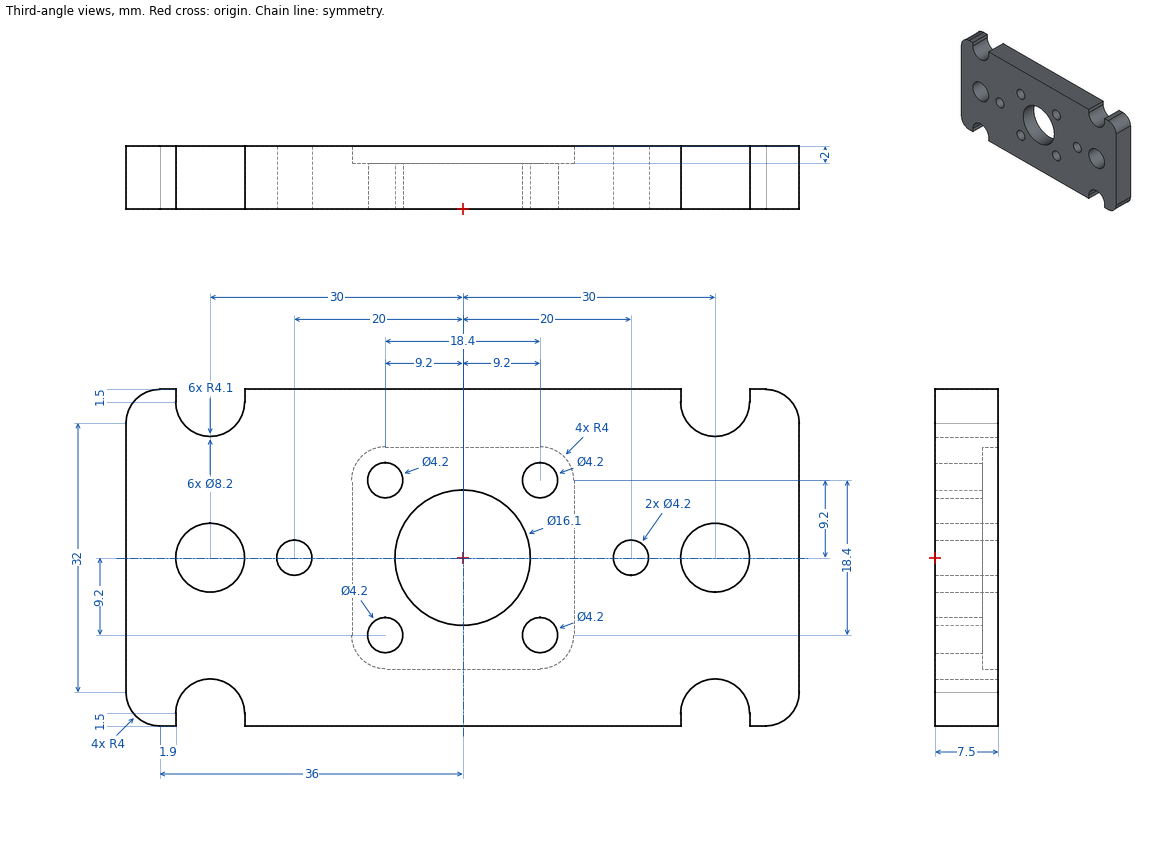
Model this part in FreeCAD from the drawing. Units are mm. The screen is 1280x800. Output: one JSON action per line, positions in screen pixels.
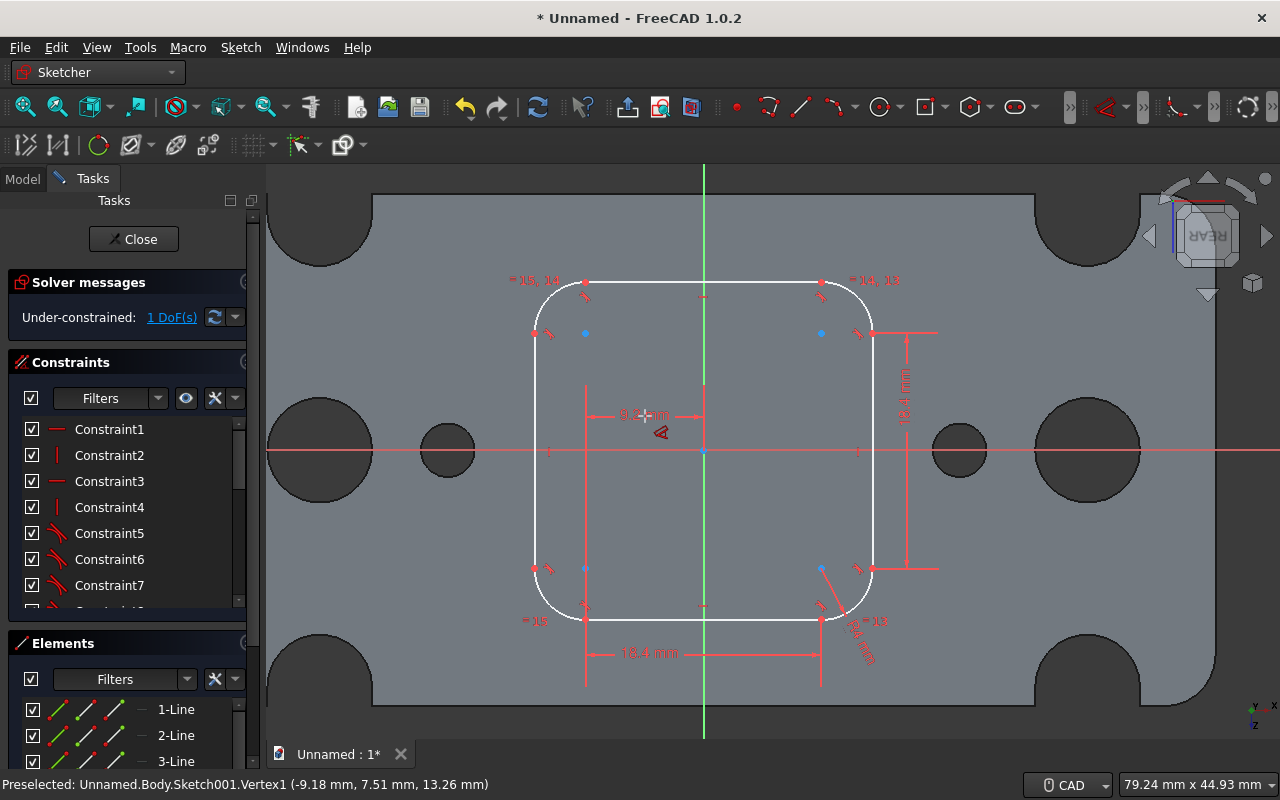
{"action": "left_click", "coordinate": [873, 569]}
{"action": "left_click", "coordinate": [907, 510]}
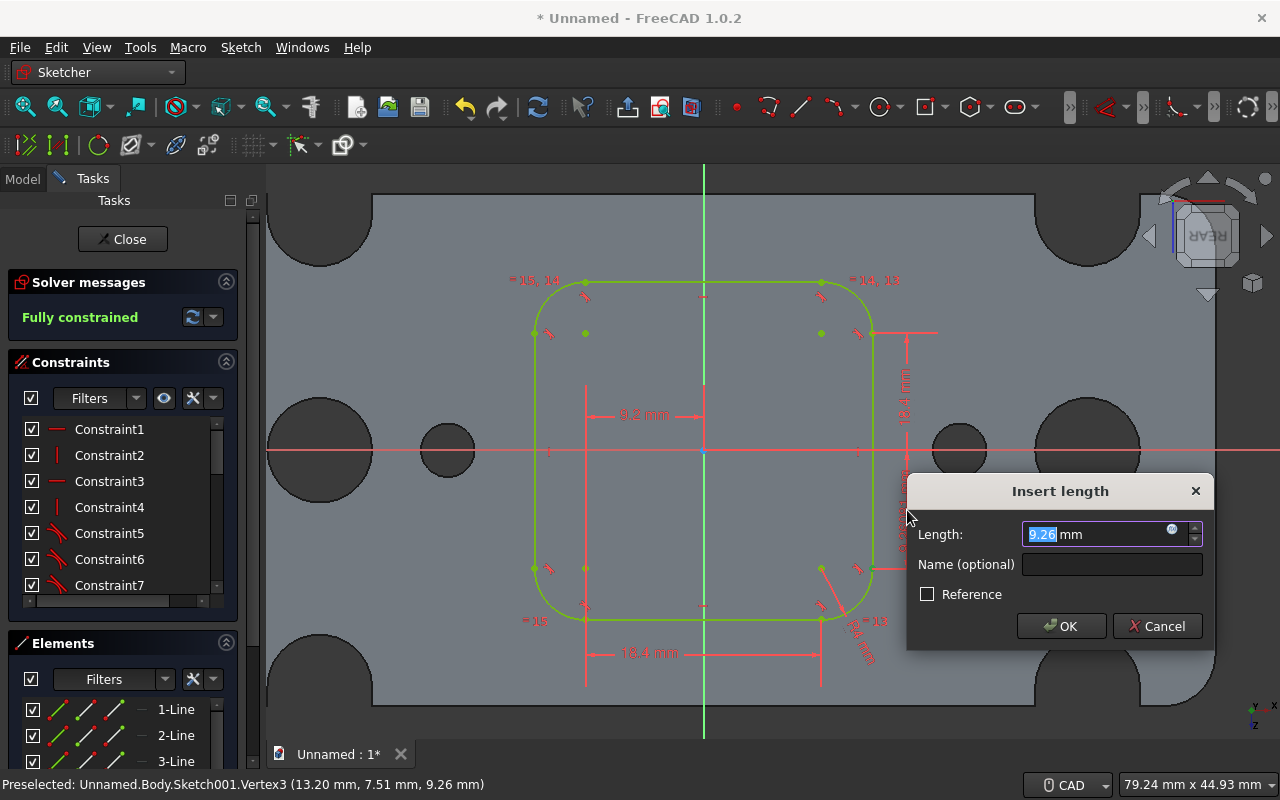
{"action": "type", "text": "9.2"}
{"action": "key", "text": "Return"}
{"action": "key", "text": "Escape"}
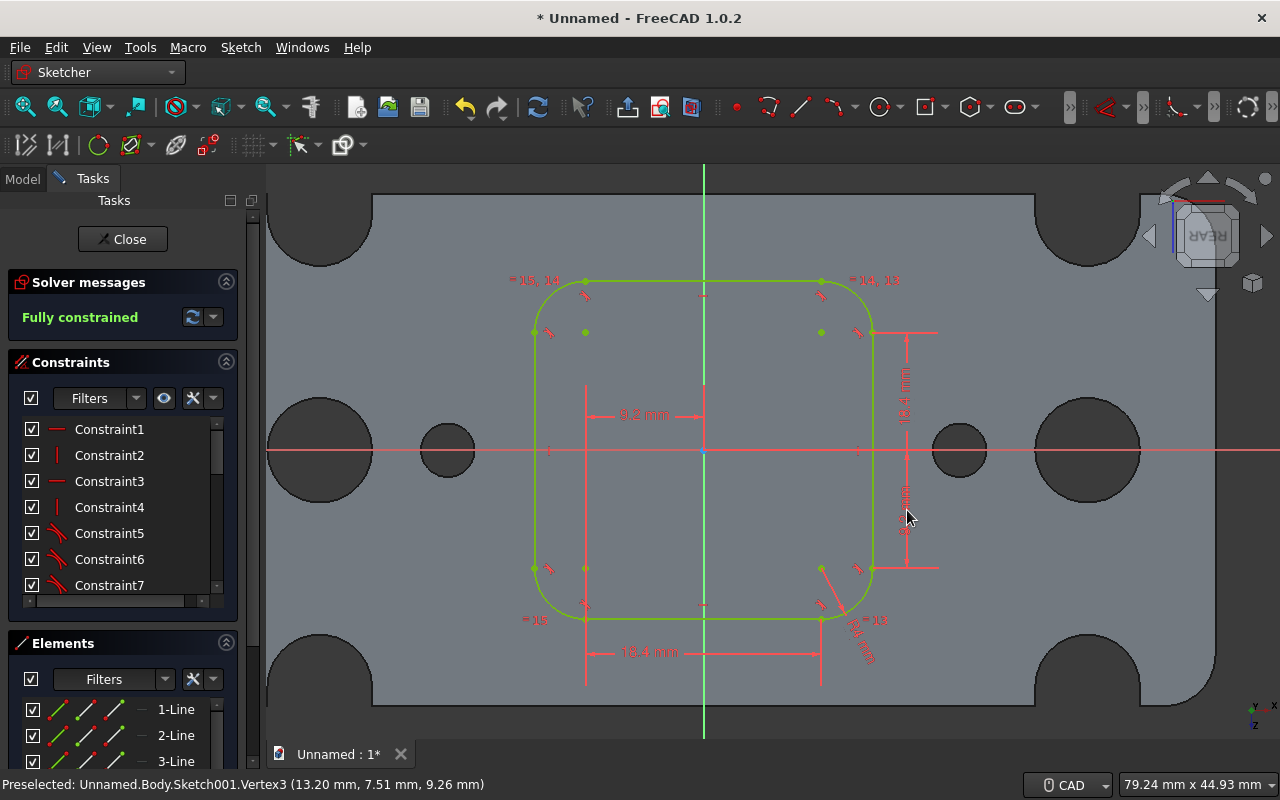
{"action": "left_click", "coordinate": [123, 239]}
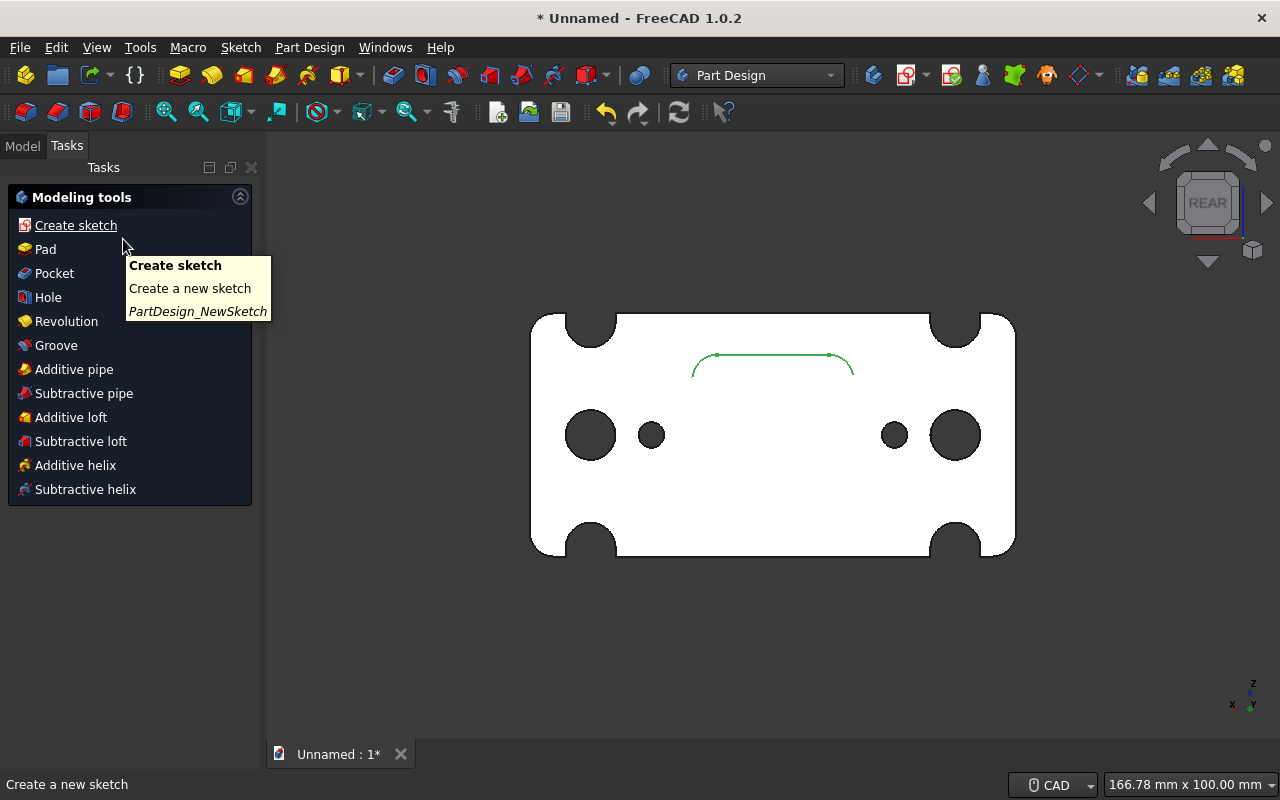
{"action": "left_click", "coordinate": [394, 76]}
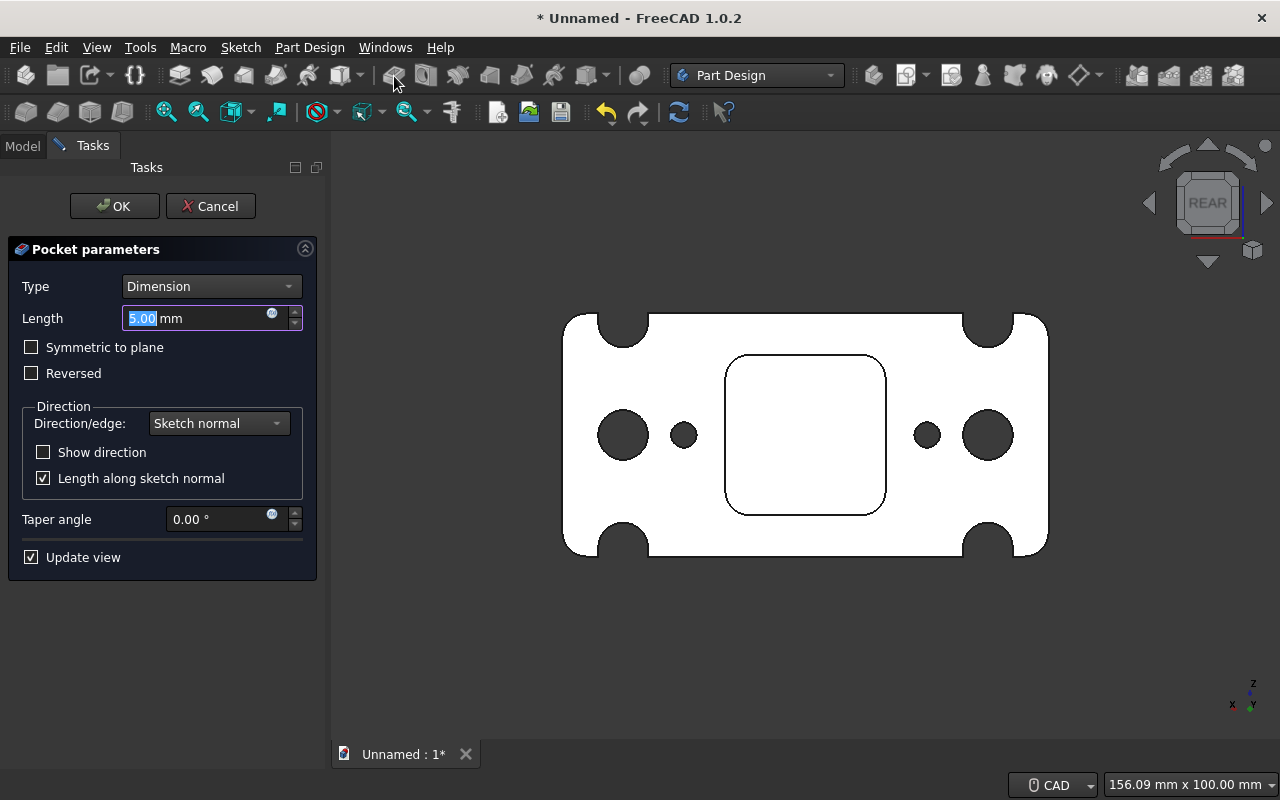
{"action": "type", "text": "2"}
{"action": "key", "text": "Tab"}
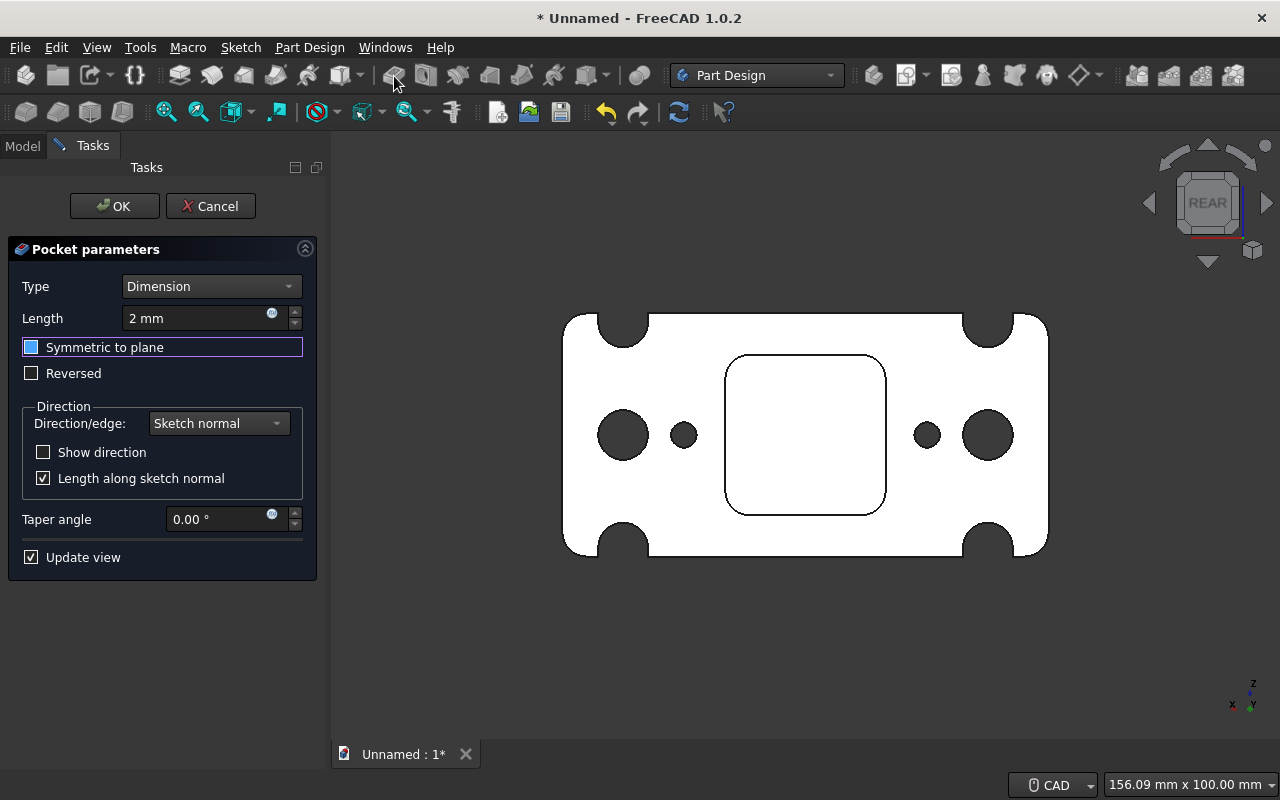
{"action": "left_click", "coordinate": [115, 206]}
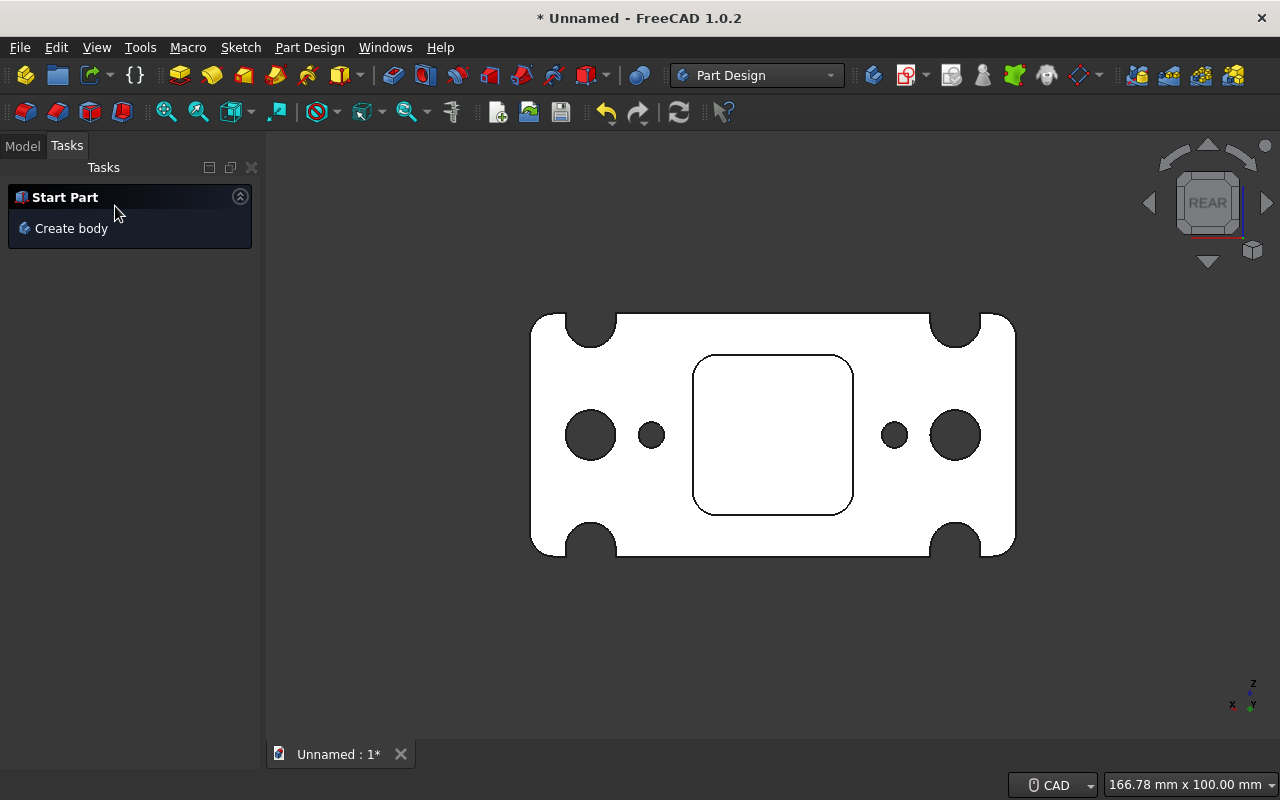
{"action": "left_click", "coordinate": [773, 434]}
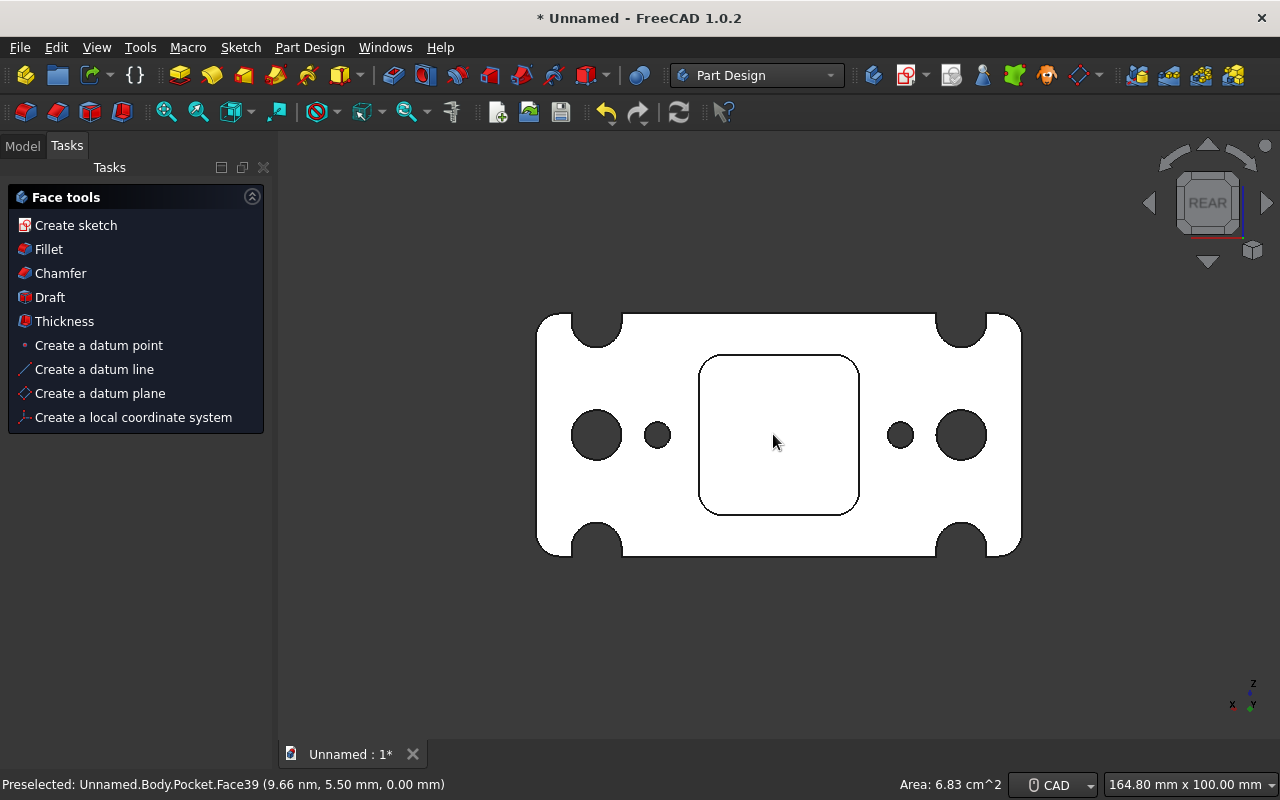
{"action": "left_click", "coordinate": [906, 76]}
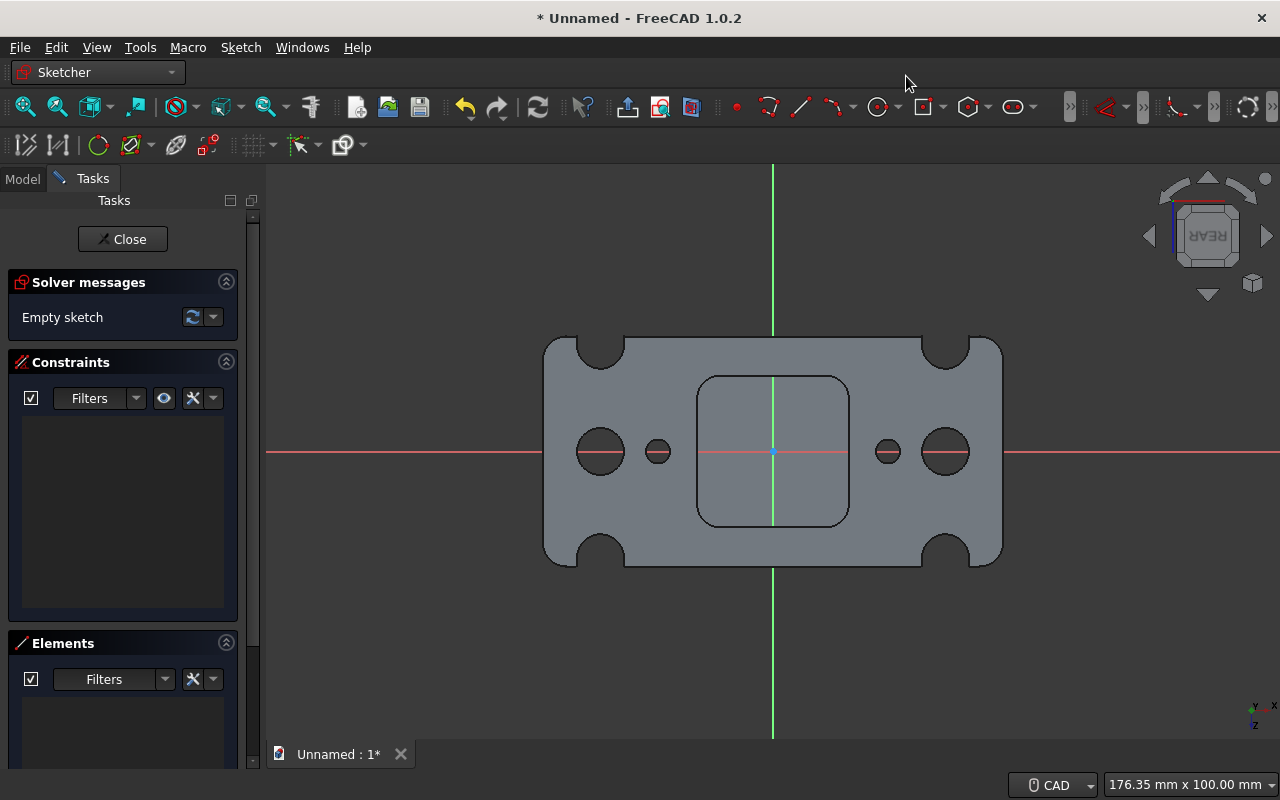
{"action": "left_click", "coordinate": [692, 108]}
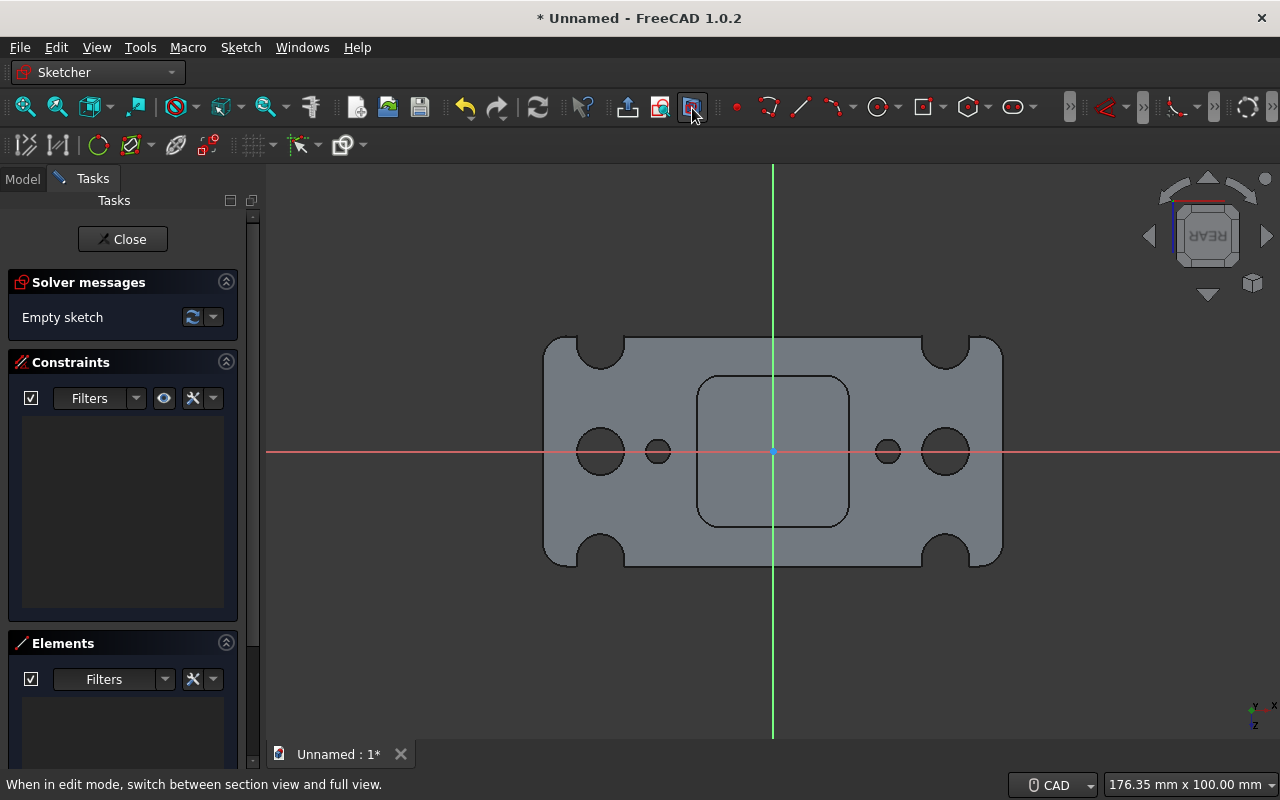
{"action": "scroll", "coordinate": [795, 451], "scroll_direction": "up", "scroll_amount": 7}